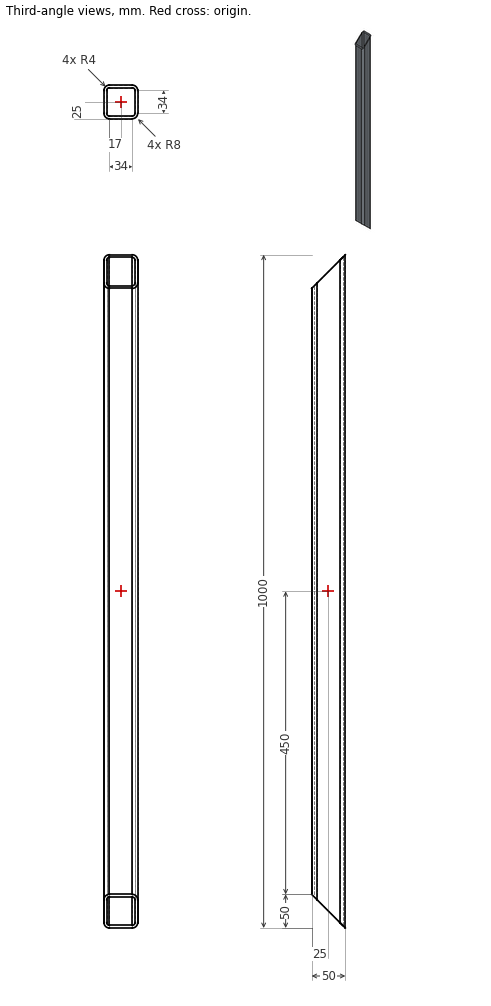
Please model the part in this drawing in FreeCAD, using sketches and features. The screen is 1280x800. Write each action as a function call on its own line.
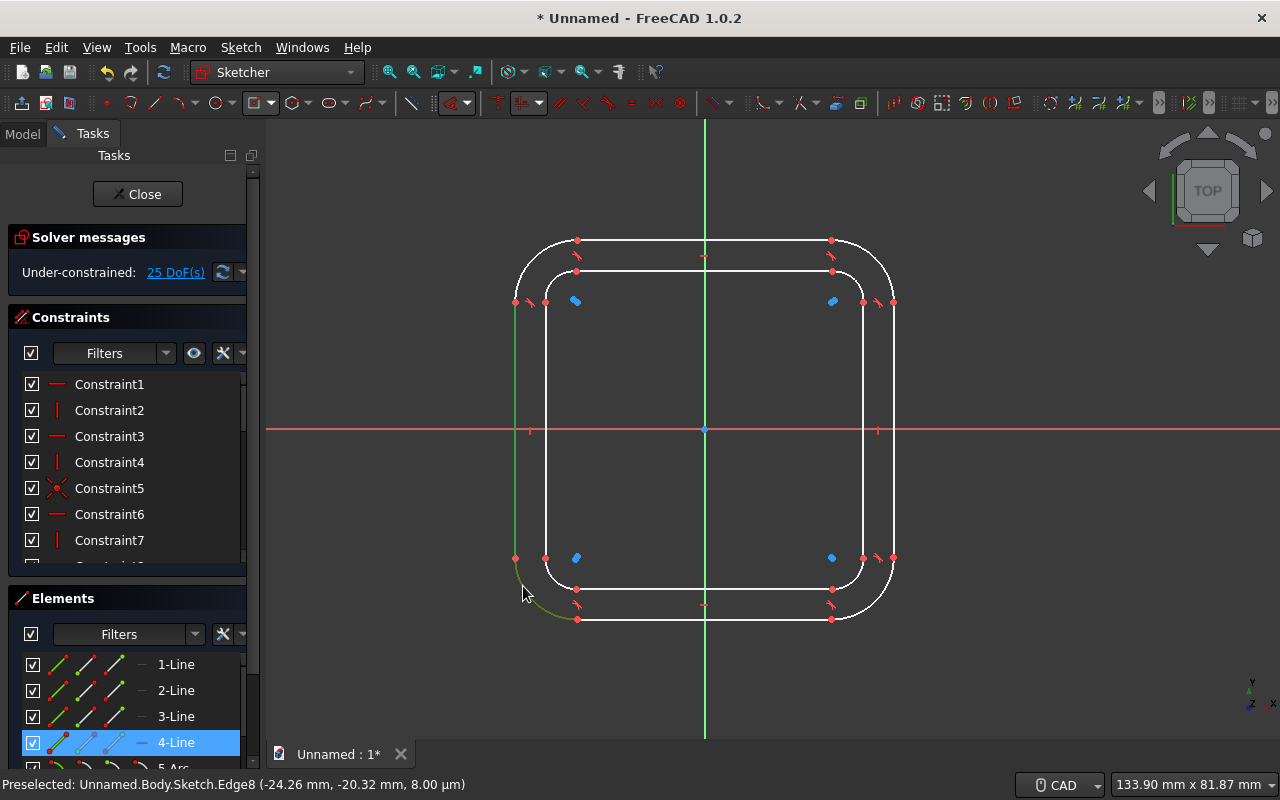
click(608, 104)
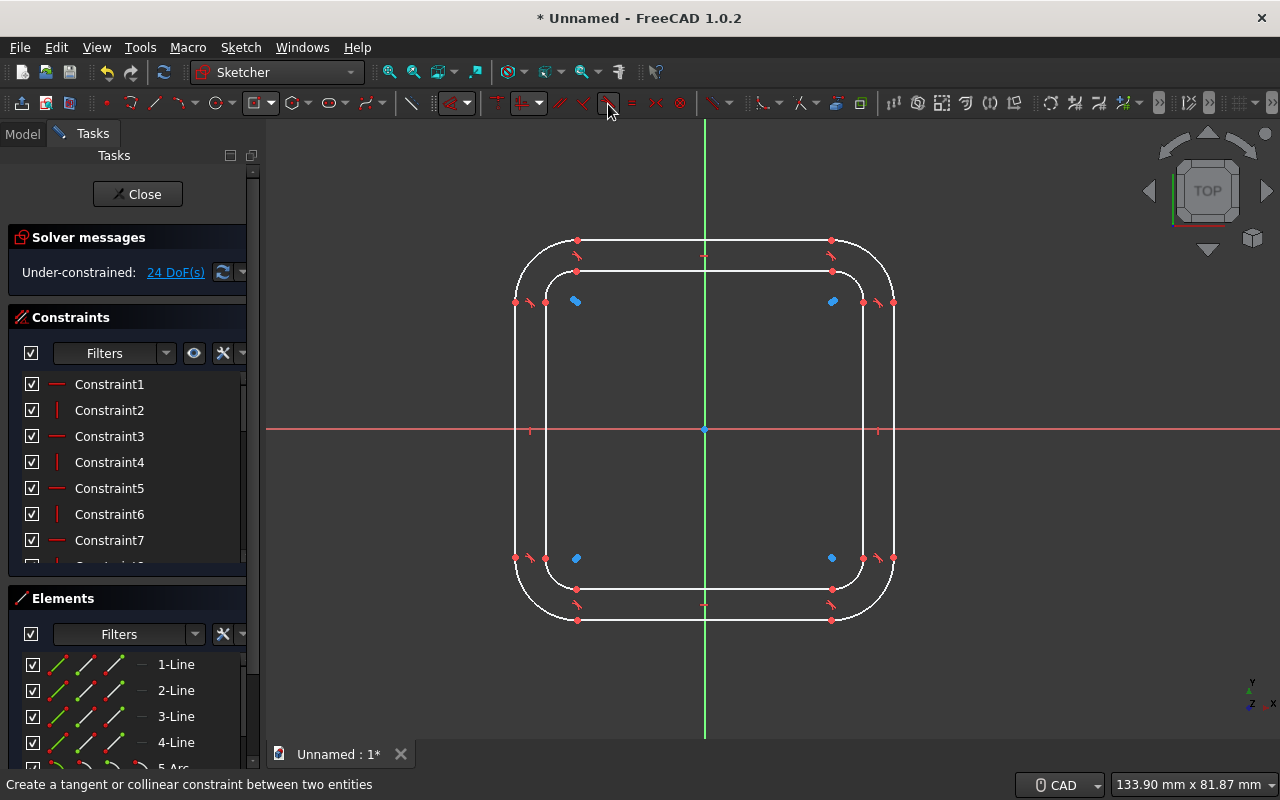
click(653, 271)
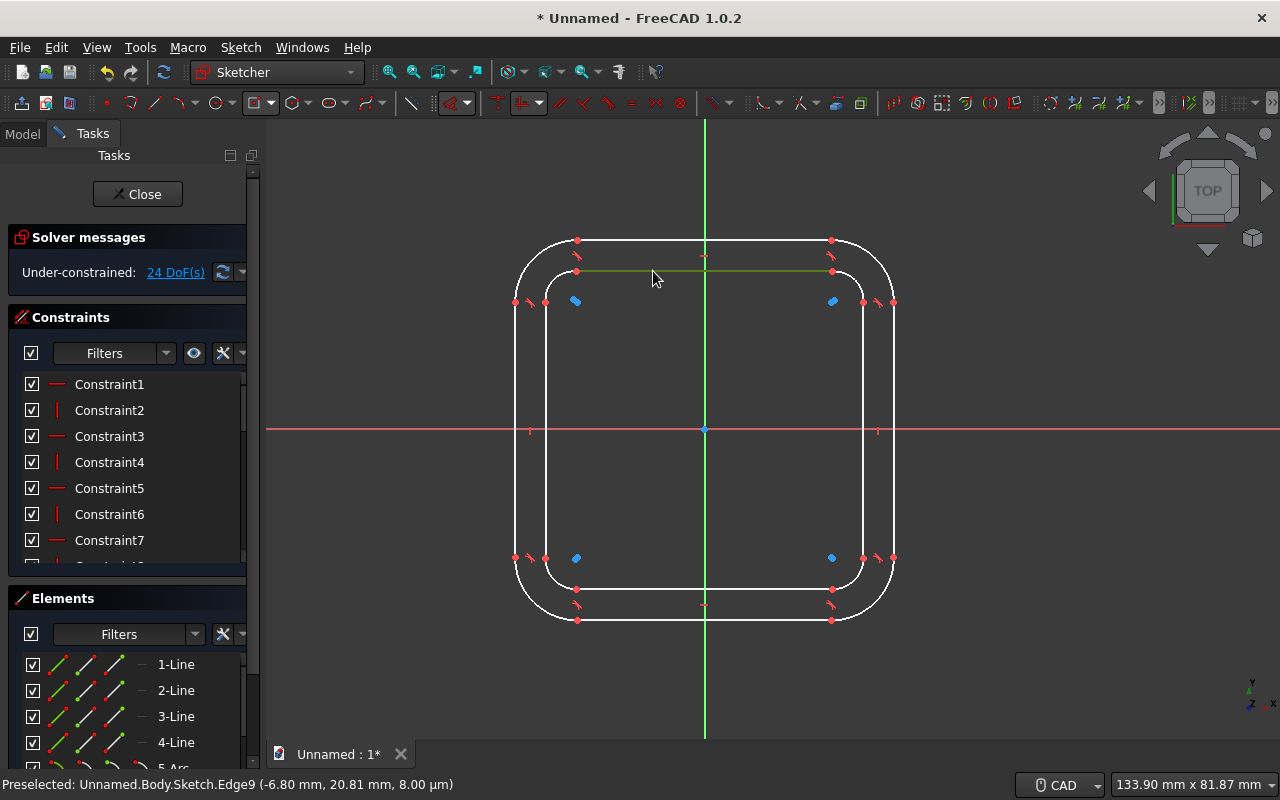
click(861, 288)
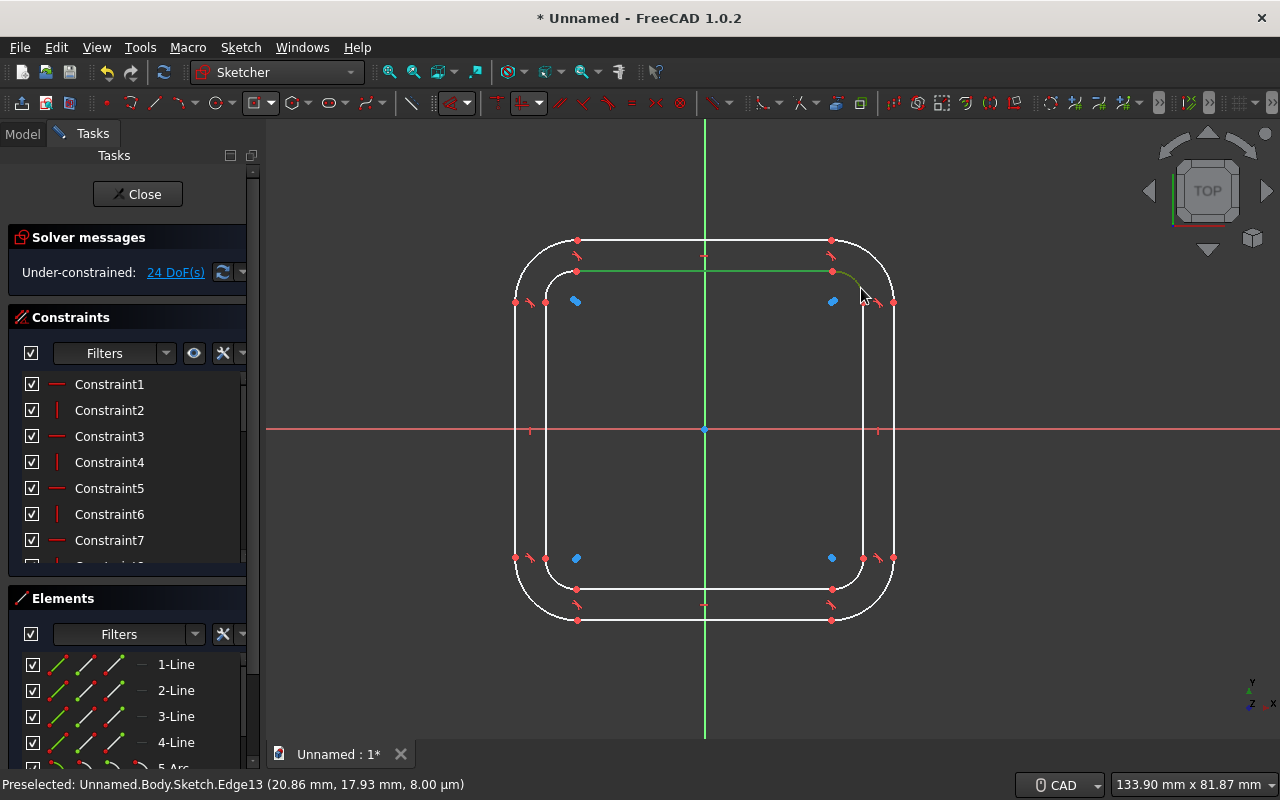
key(t)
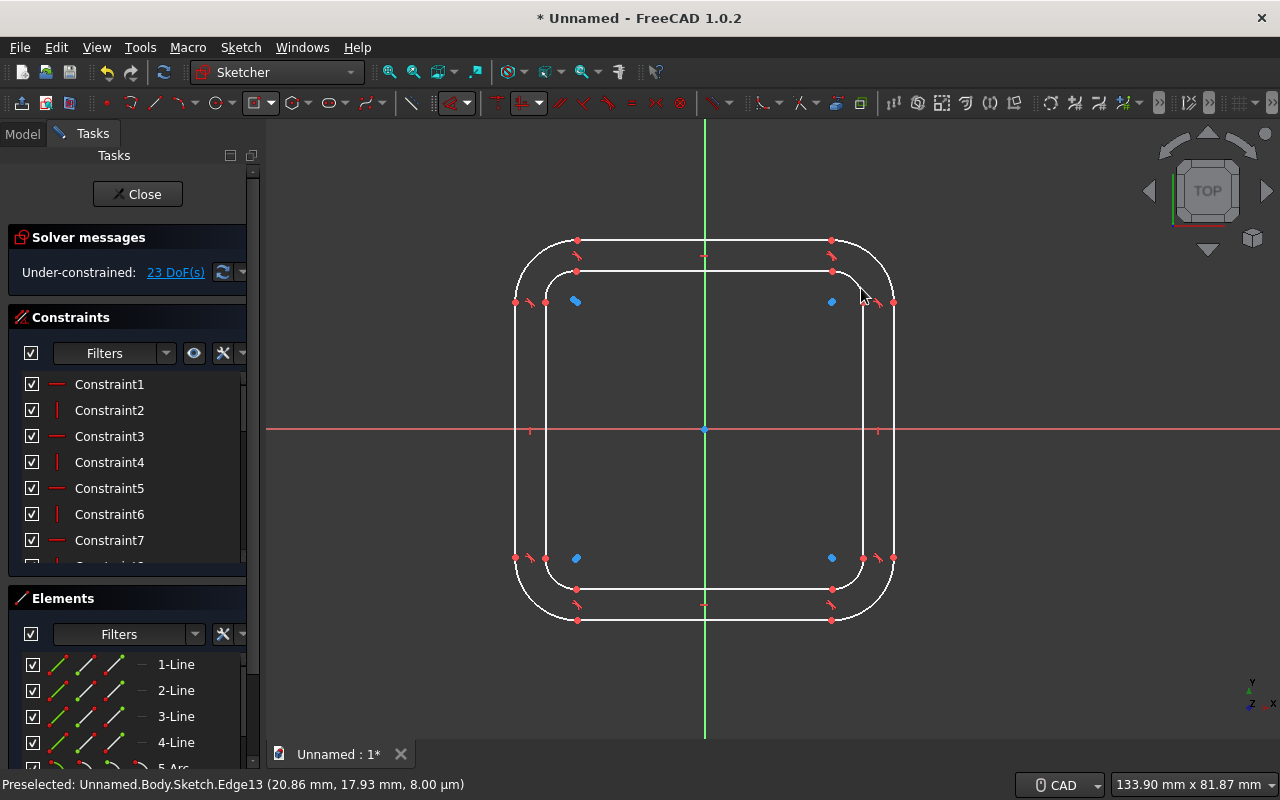
click(653, 271)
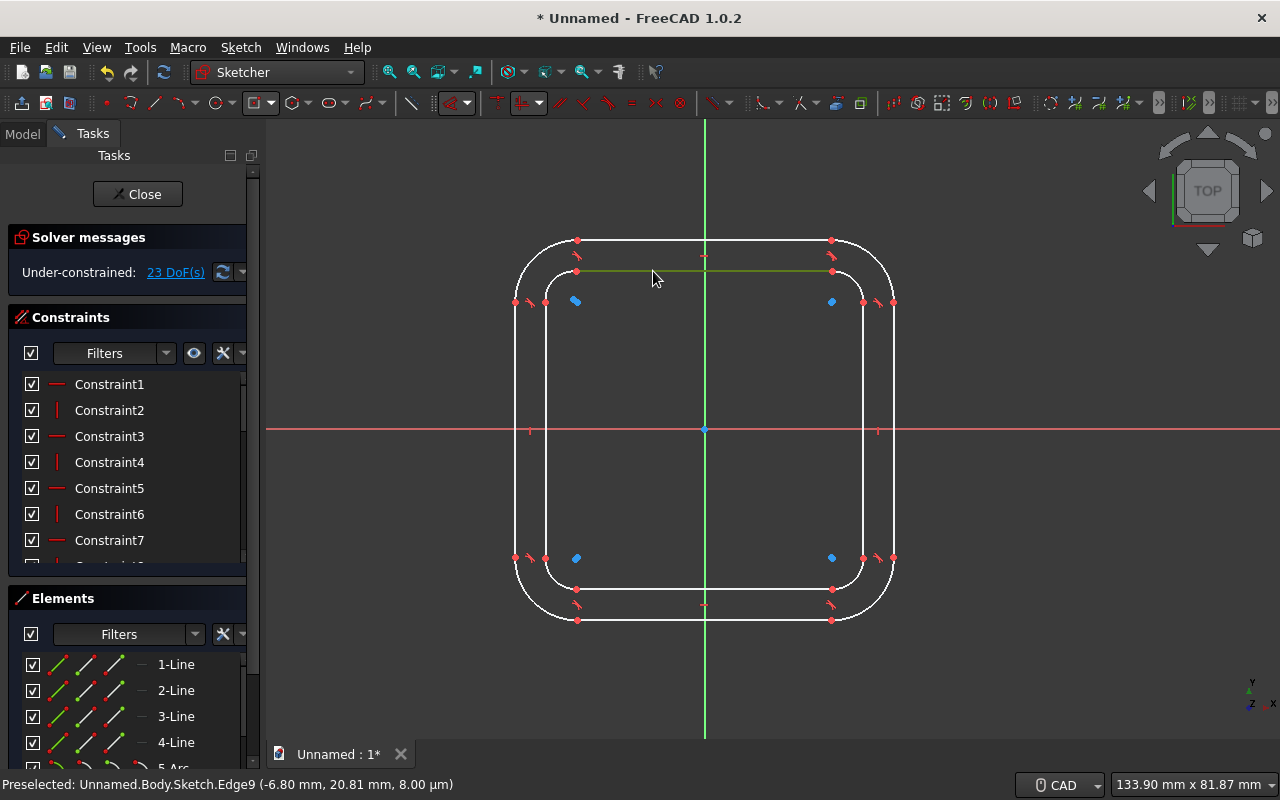
click(562, 274)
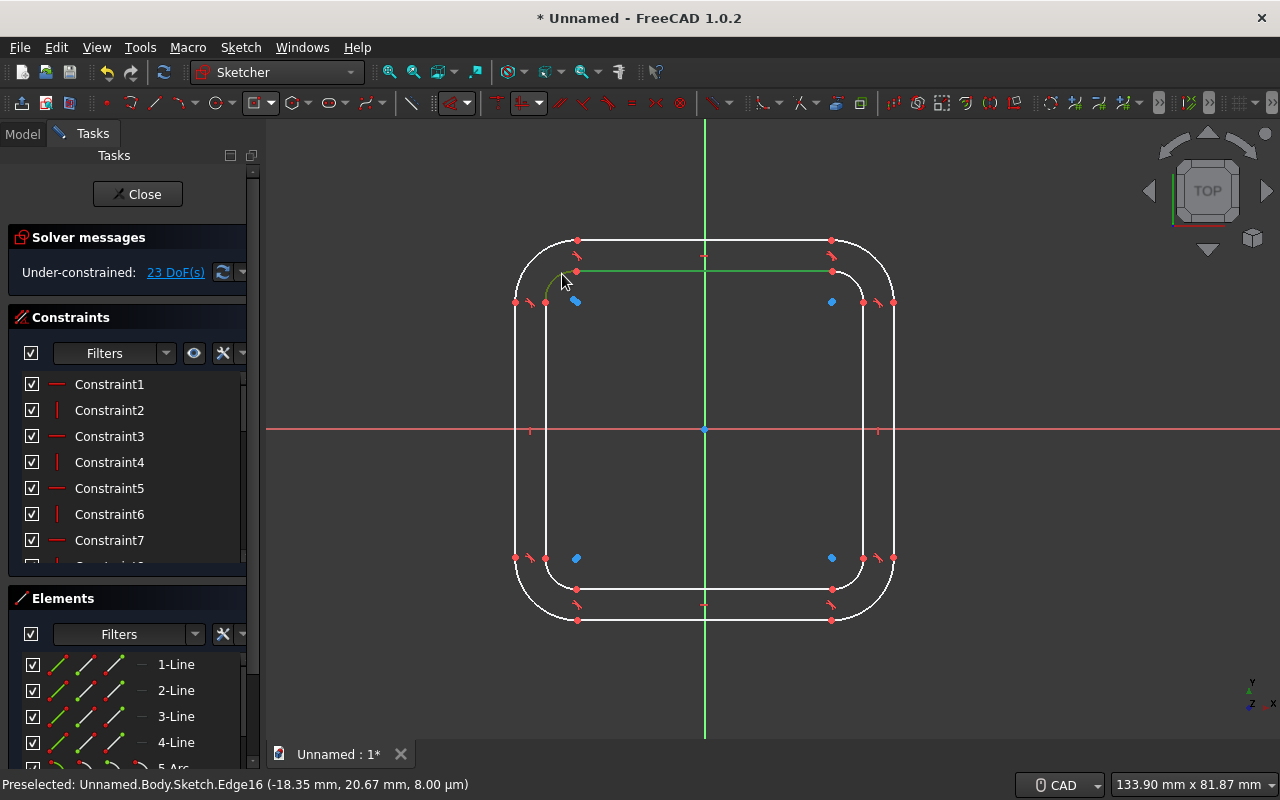
key(t)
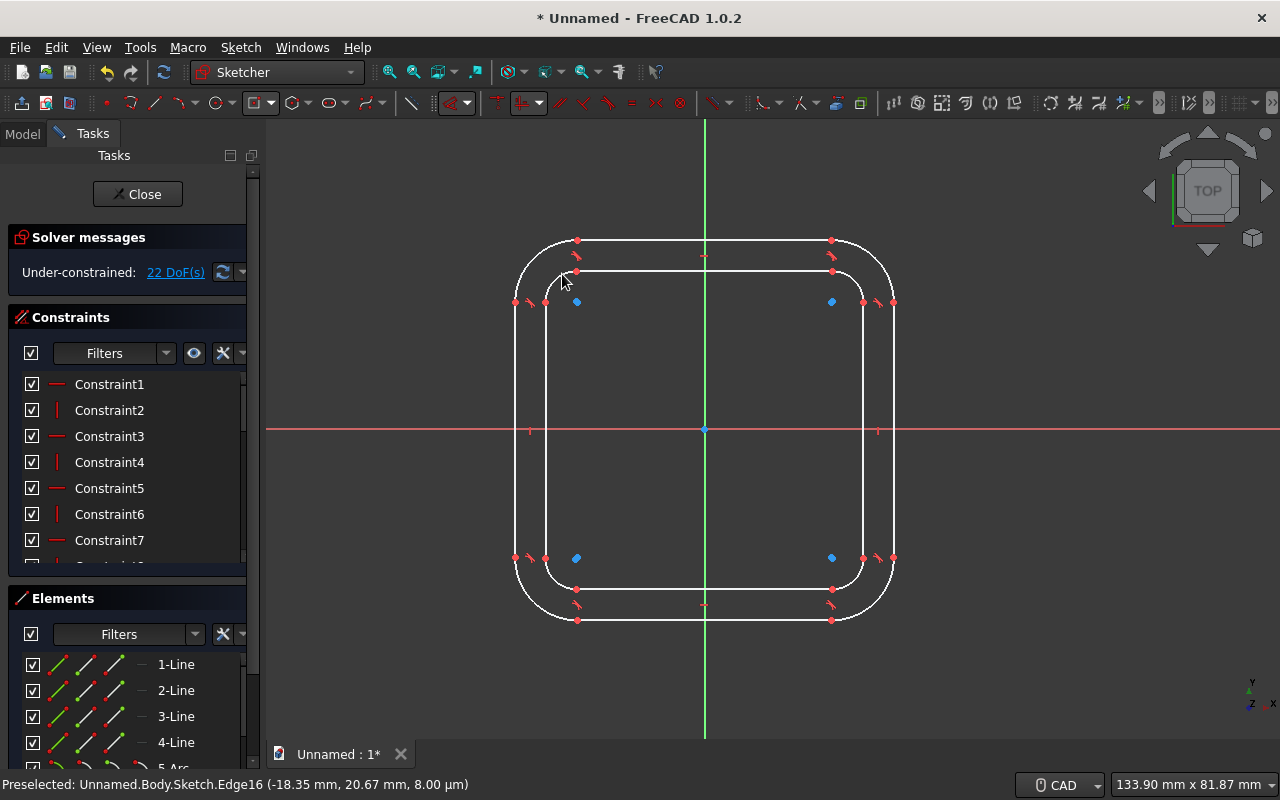
click(863, 379)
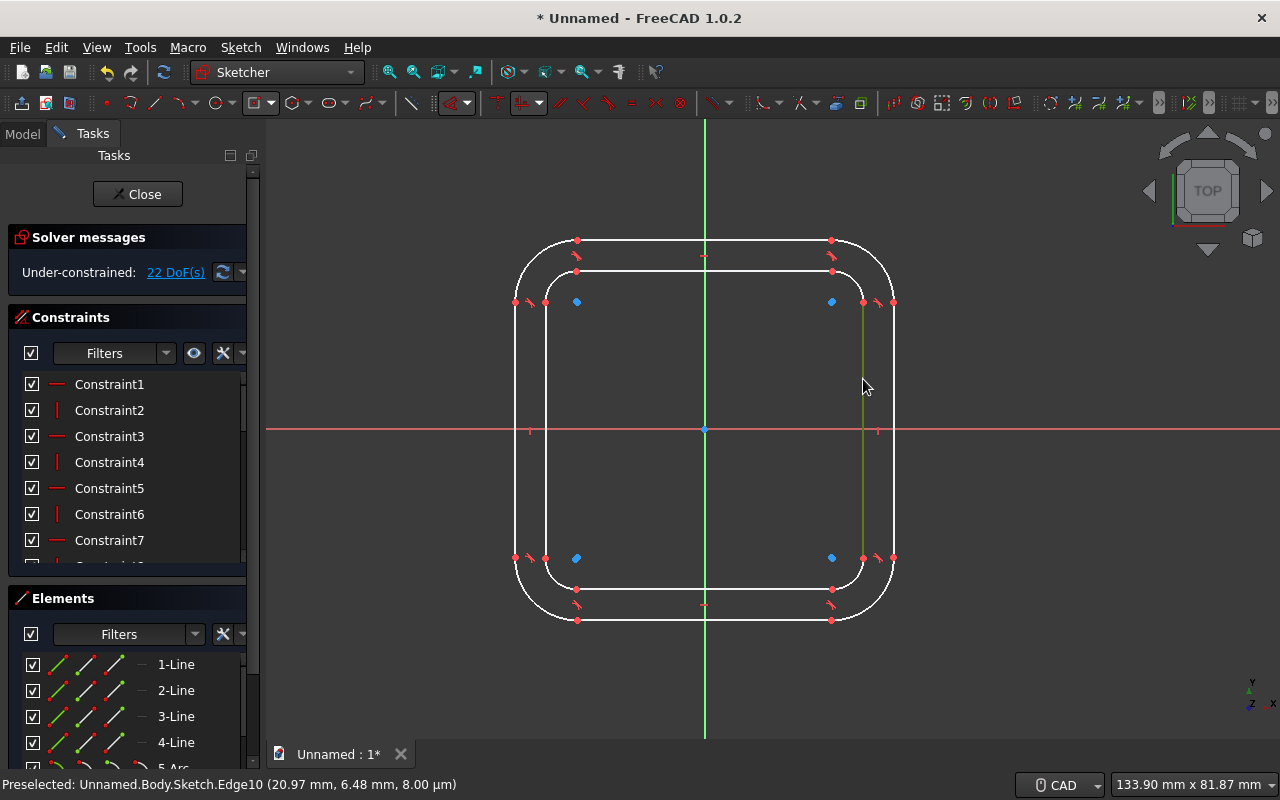
click(860, 288)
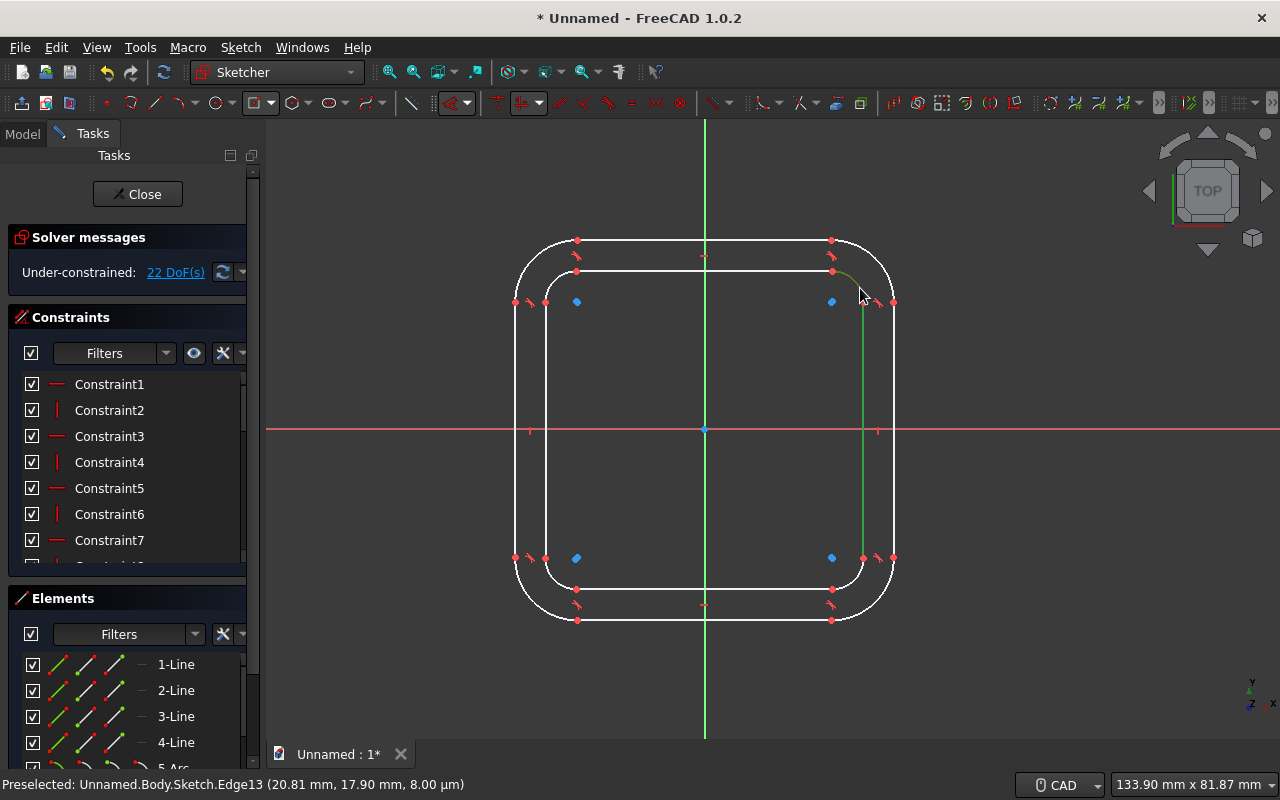
key(t)